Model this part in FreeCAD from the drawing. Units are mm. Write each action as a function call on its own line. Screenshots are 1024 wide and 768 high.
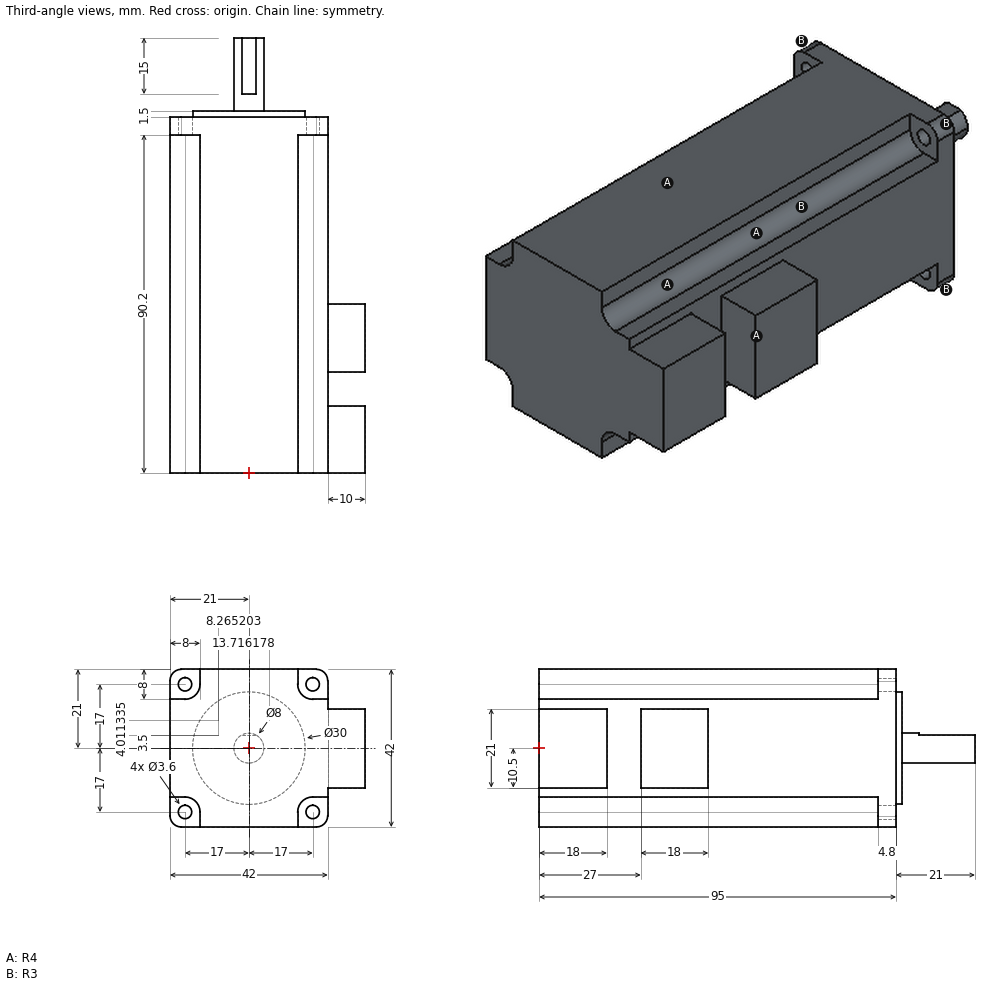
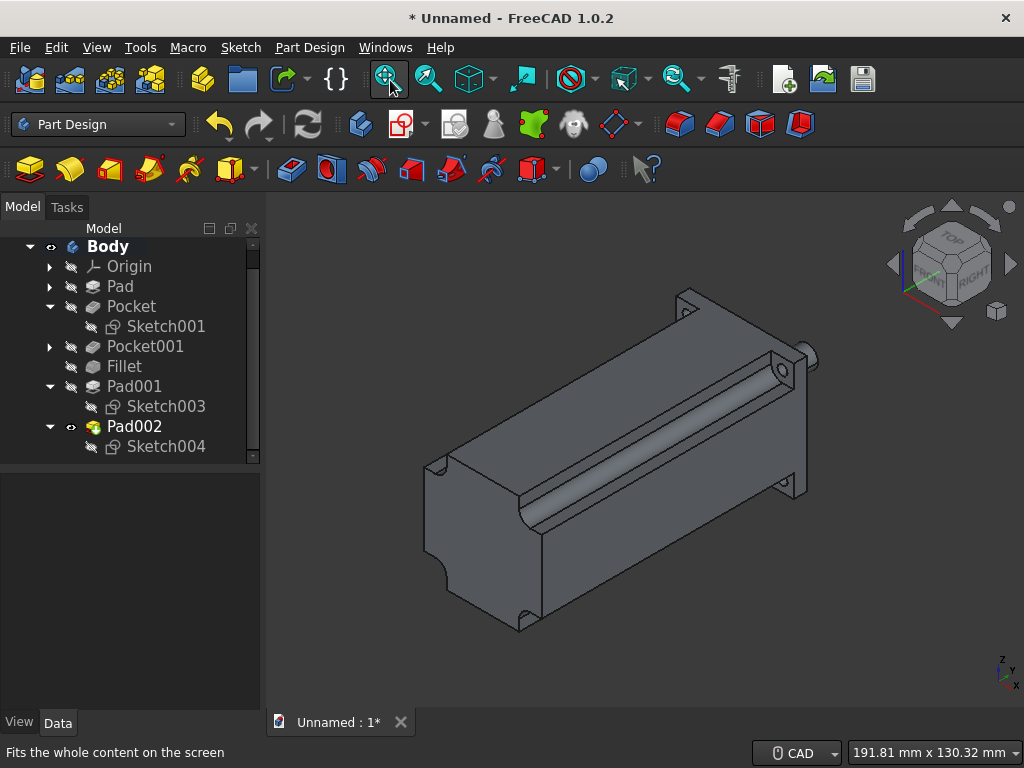
click(800, 359)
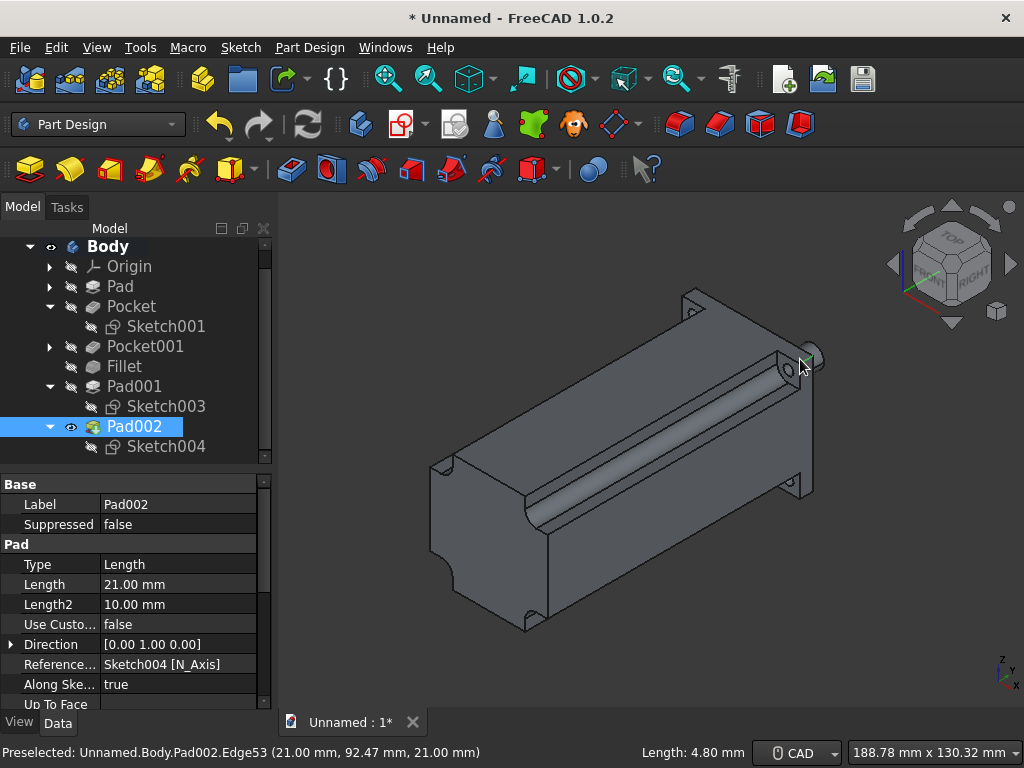
scroll(689, 291, up, 4)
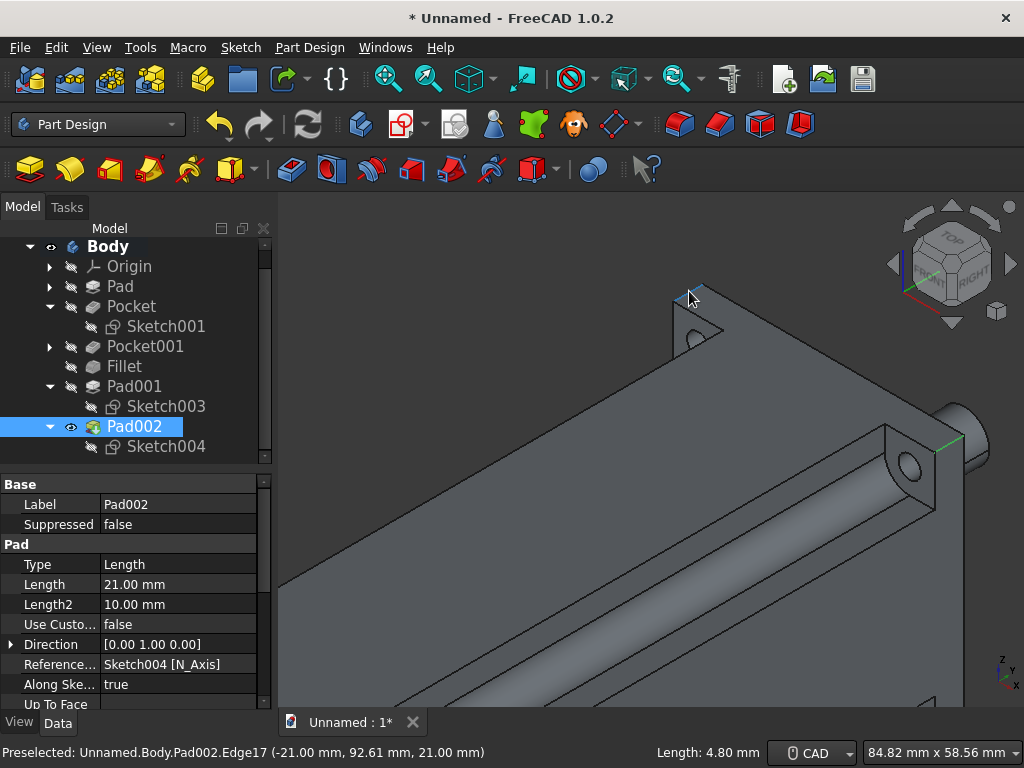
click(390, 80)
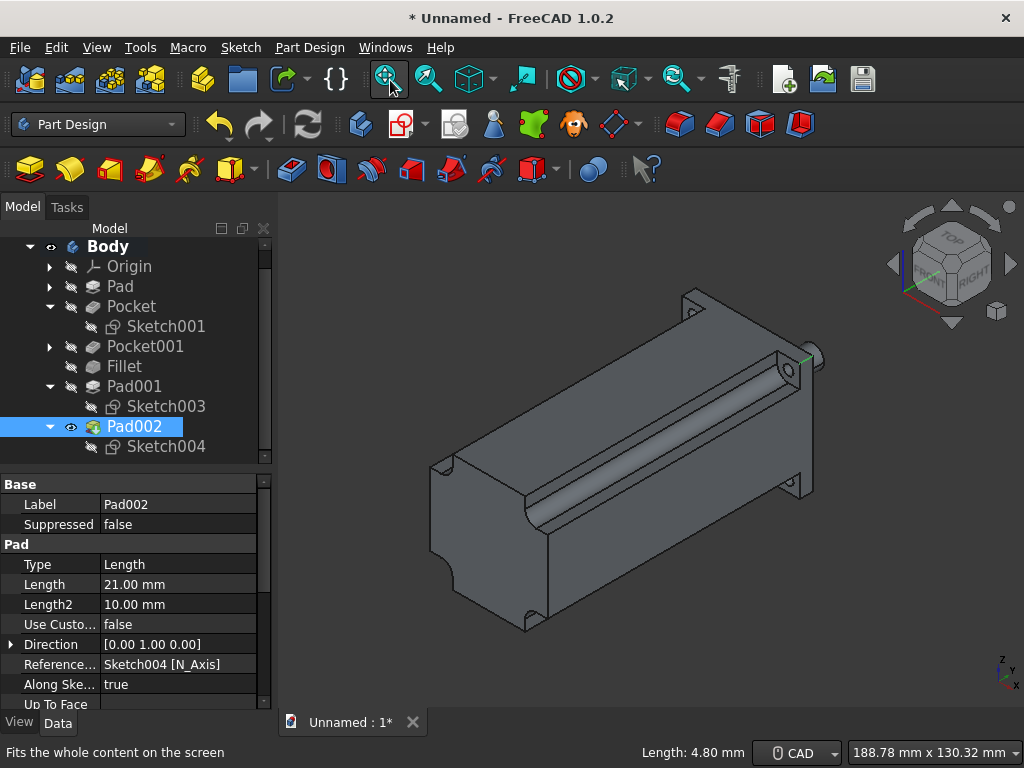
key(2)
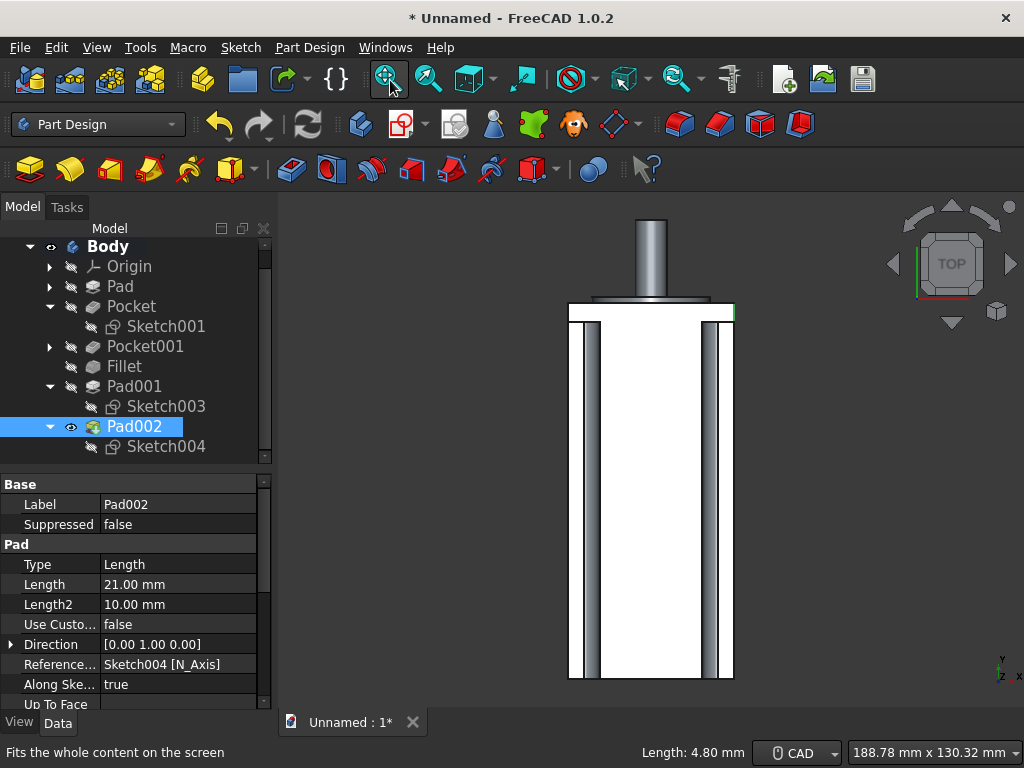
click(568, 312, ctrl)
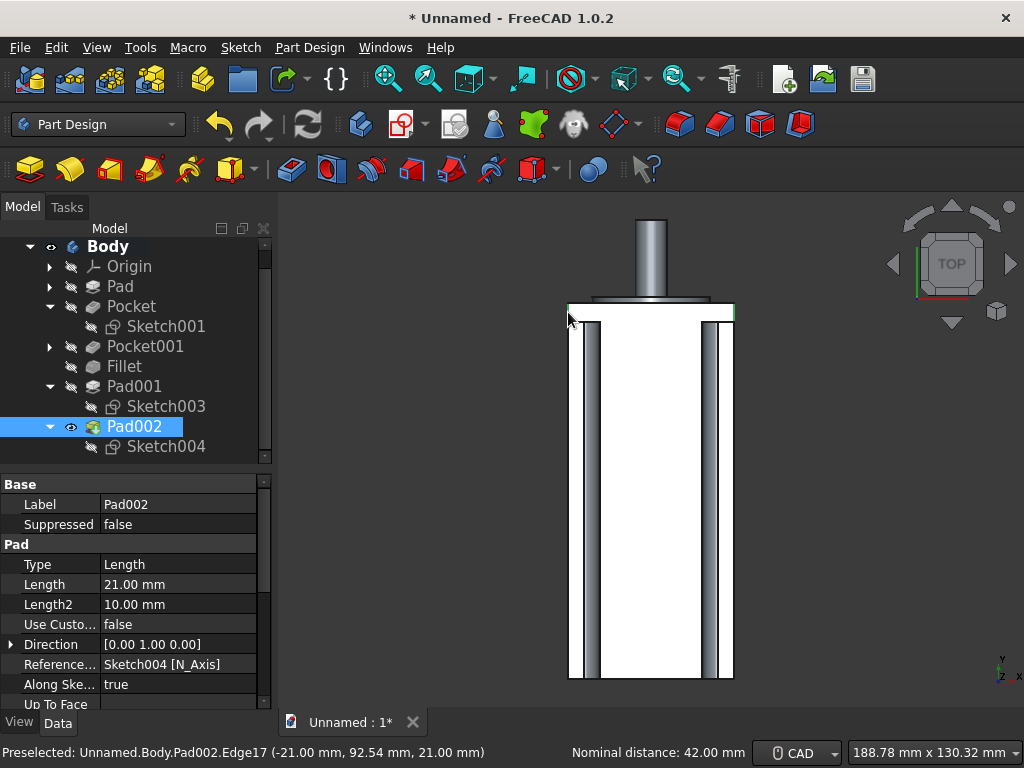
scroll(568, 312, up, 4)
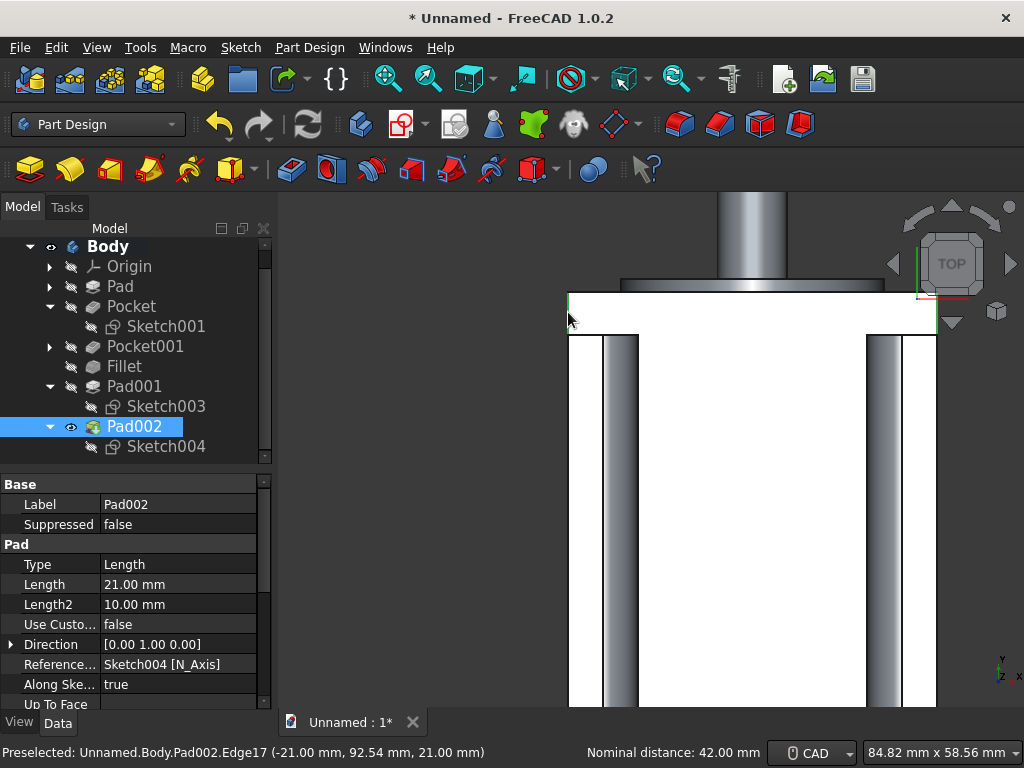
key(v)
key(f)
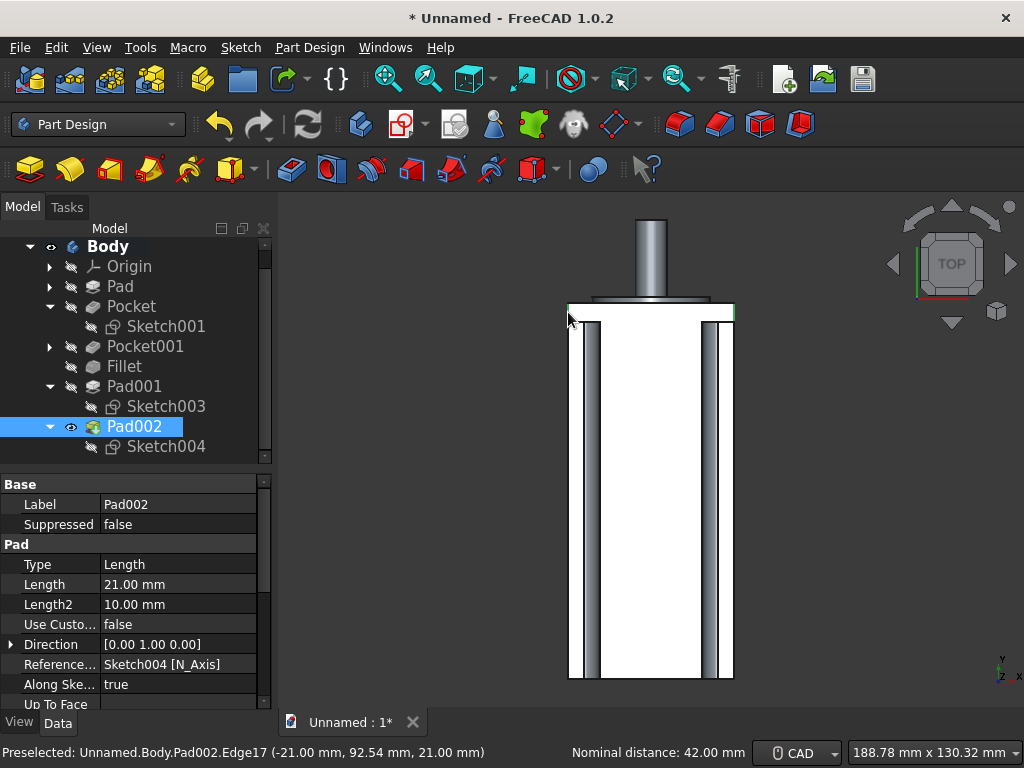
key(1)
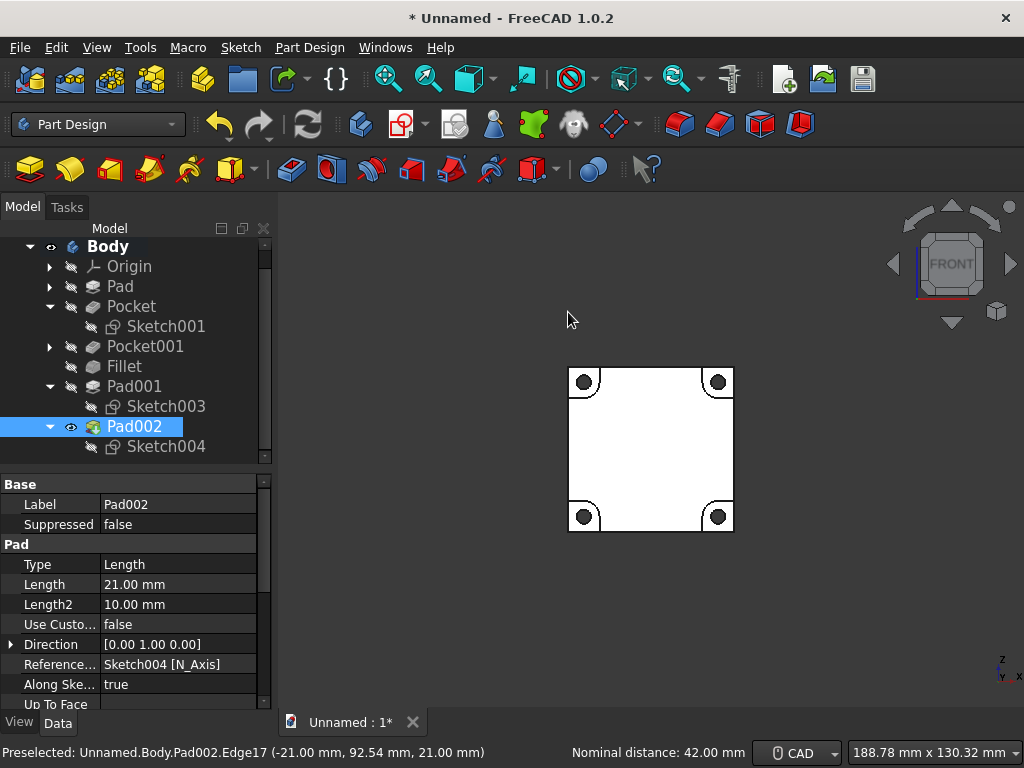
click(390, 80)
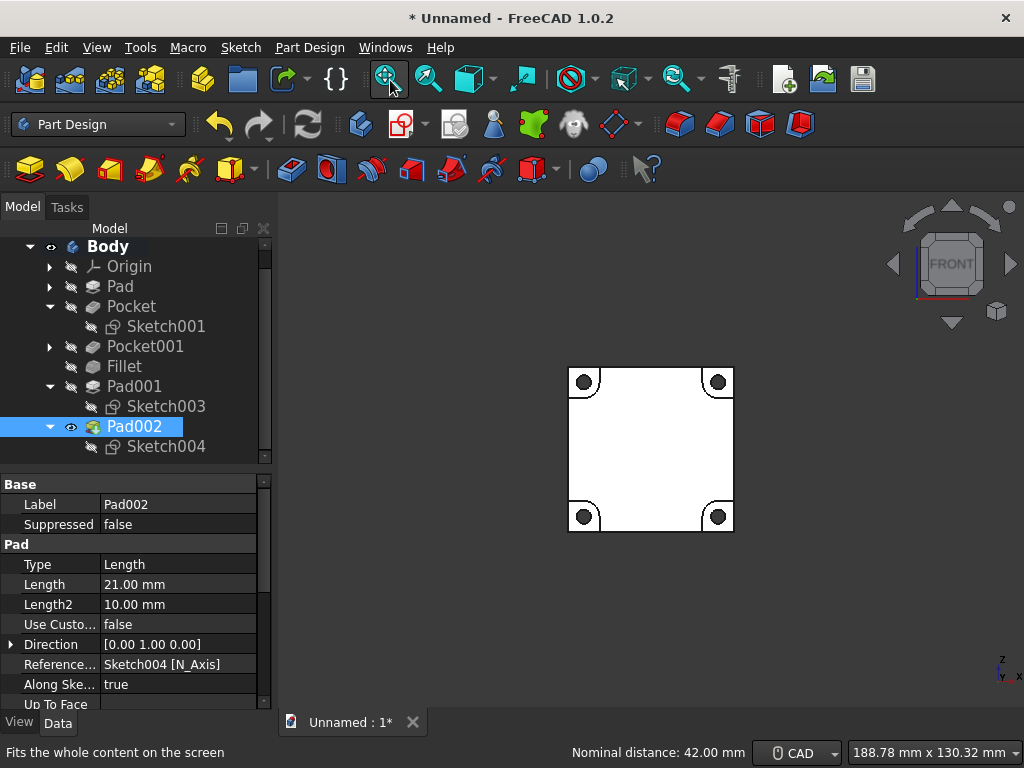
scroll(568, 531, up, 4)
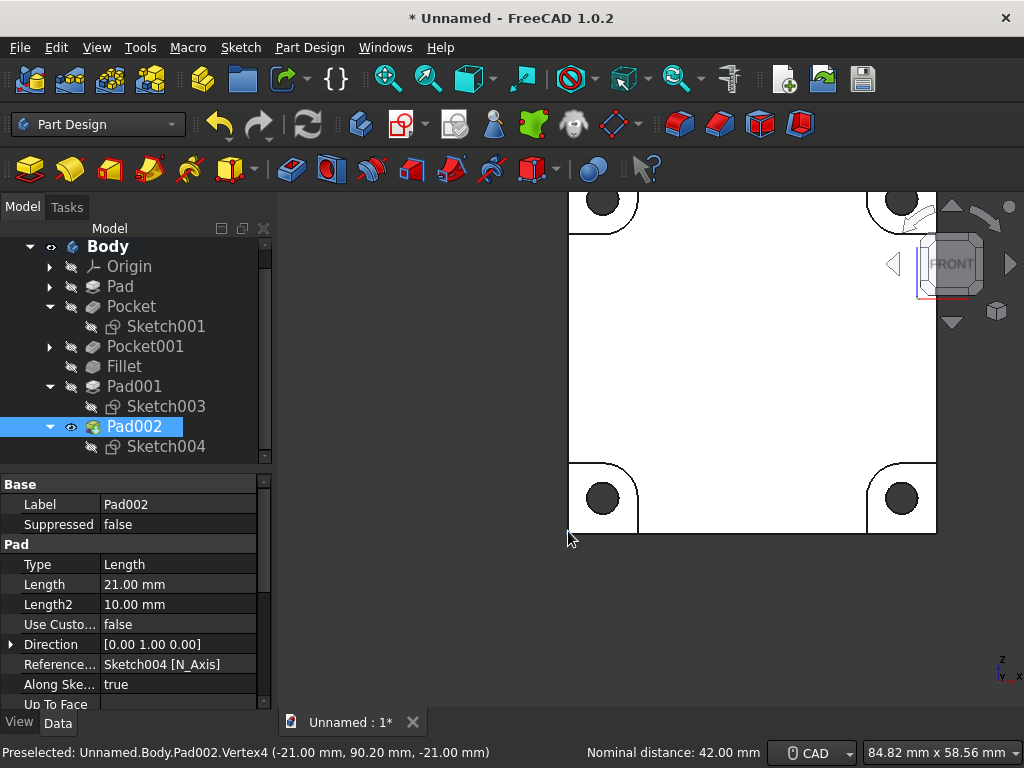
click(390, 80)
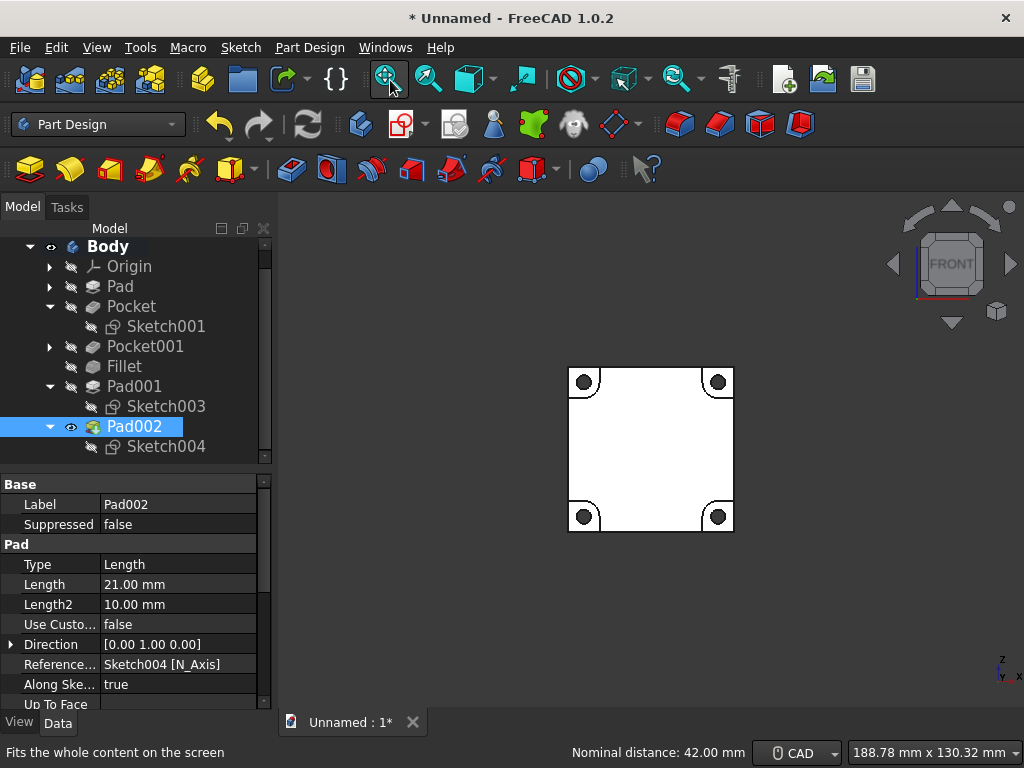
key(3)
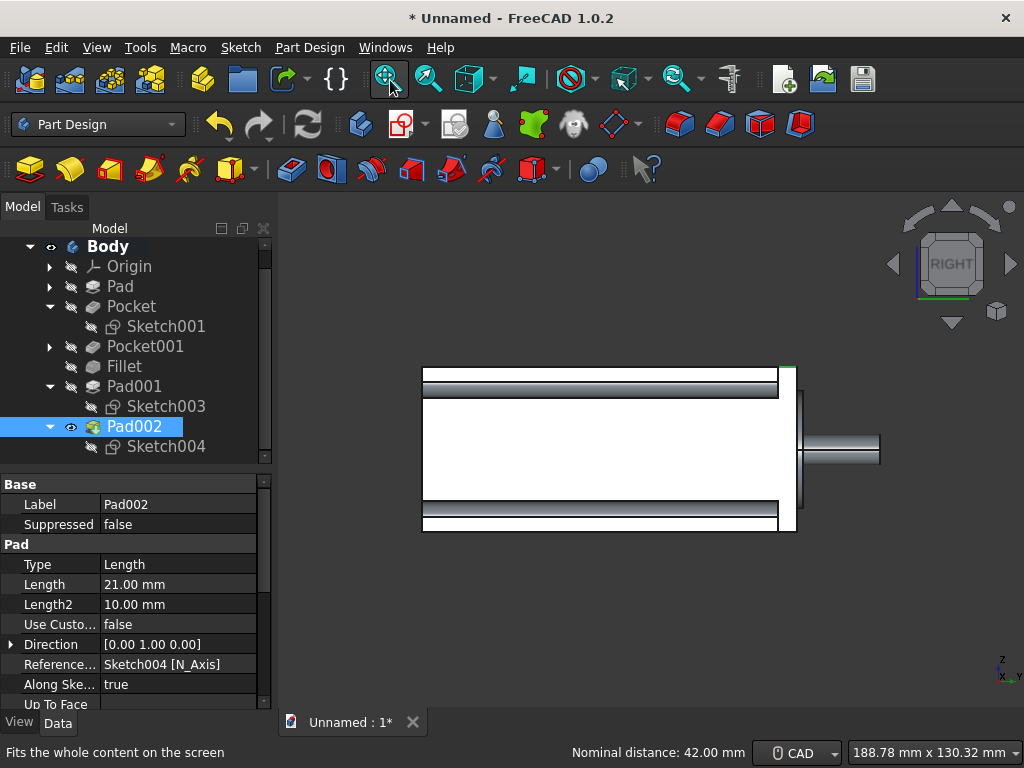
click(788, 531, ctrl)